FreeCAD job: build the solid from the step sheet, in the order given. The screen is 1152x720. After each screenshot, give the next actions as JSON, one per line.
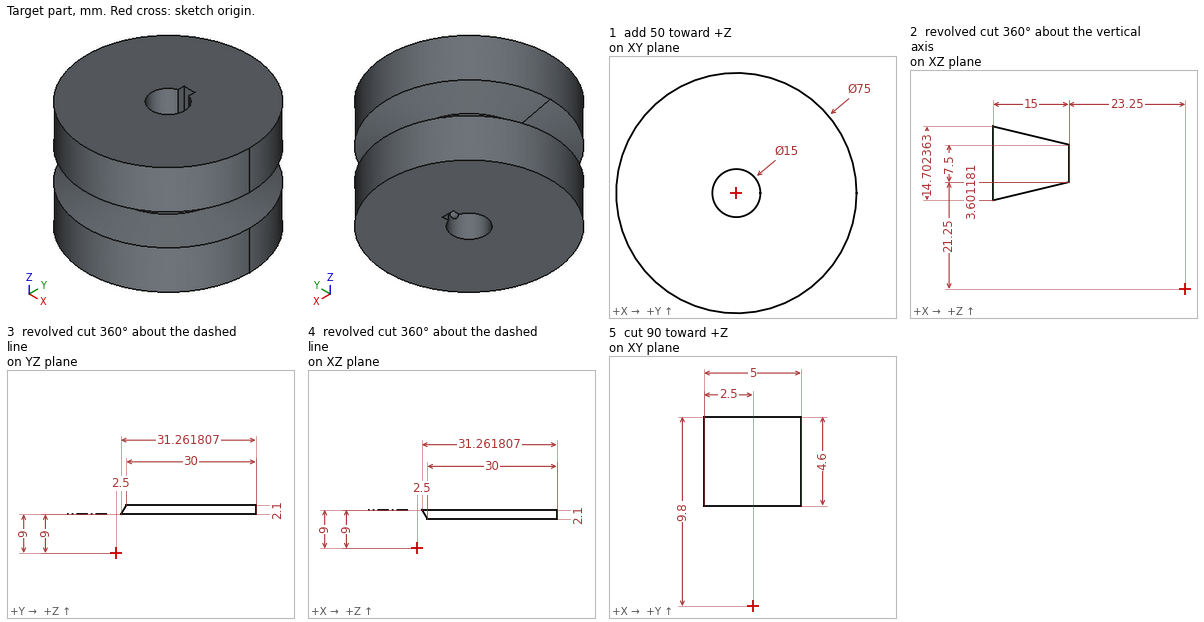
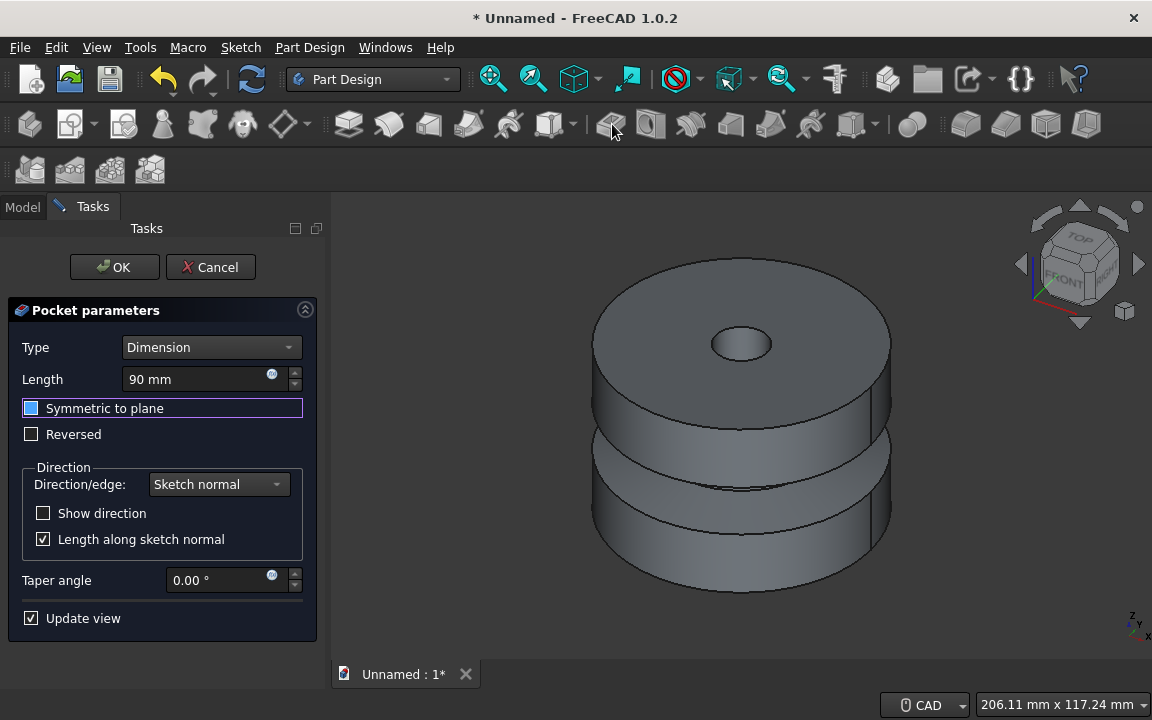
{"action": "left_click", "coordinate": [30, 434]}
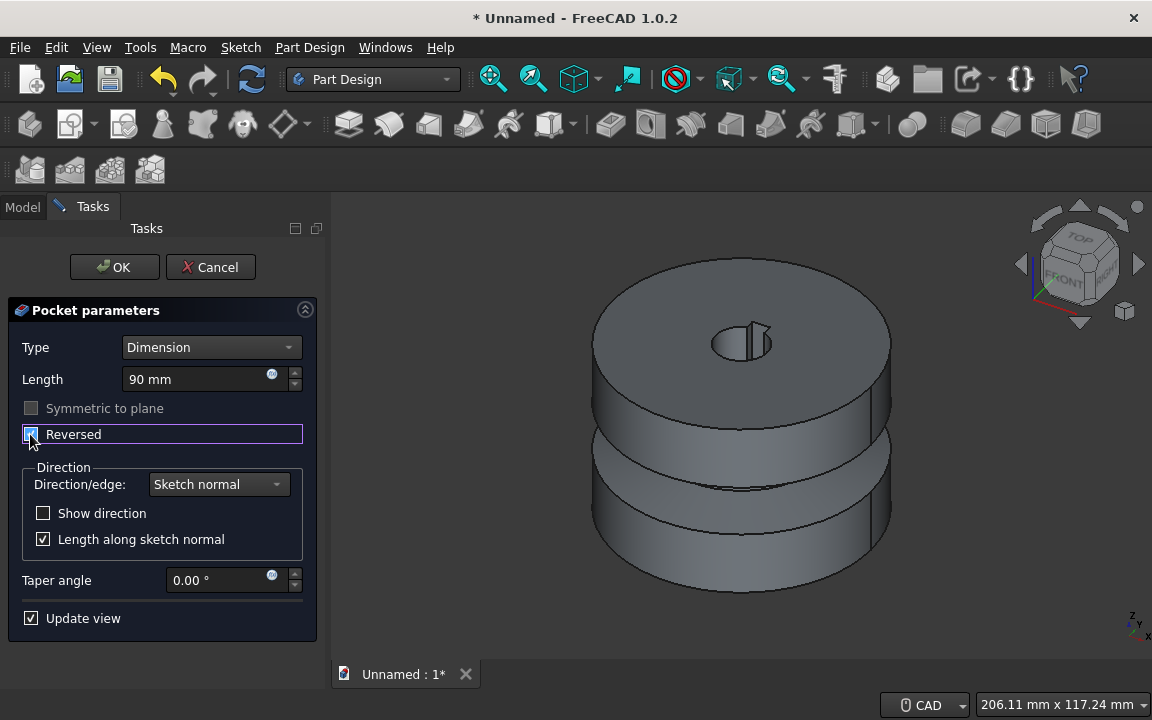
{"action": "left_click", "coordinate": [115, 267]}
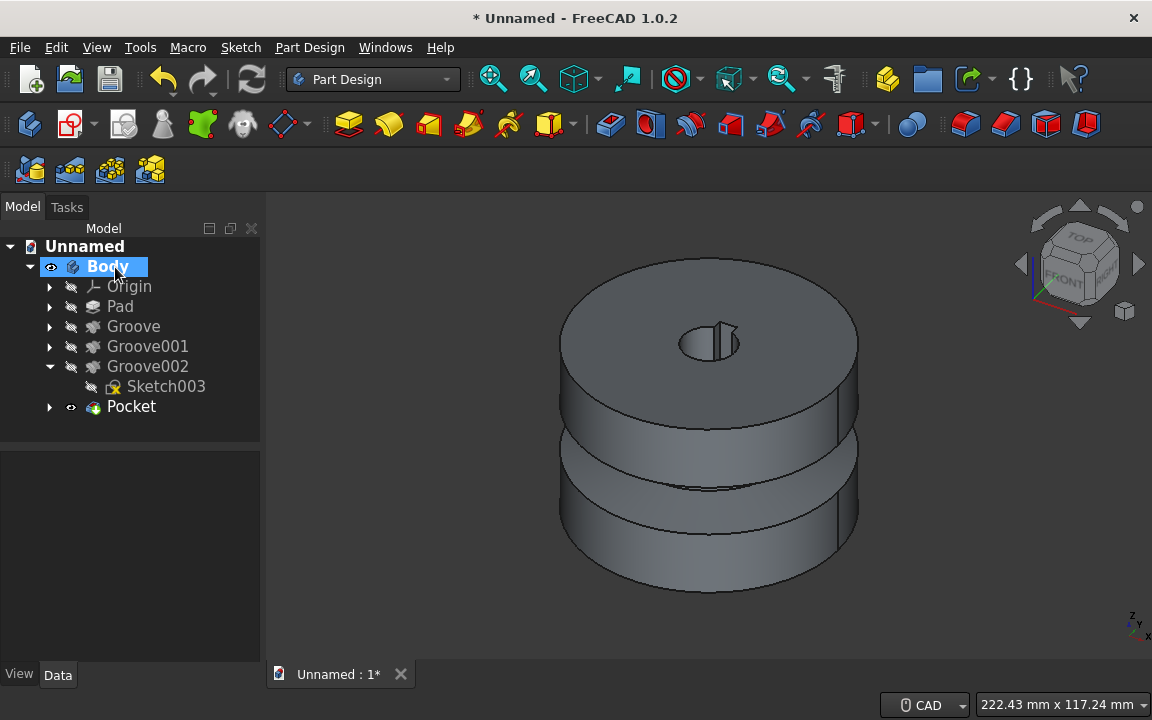
{"action": "key", "text": "0"}